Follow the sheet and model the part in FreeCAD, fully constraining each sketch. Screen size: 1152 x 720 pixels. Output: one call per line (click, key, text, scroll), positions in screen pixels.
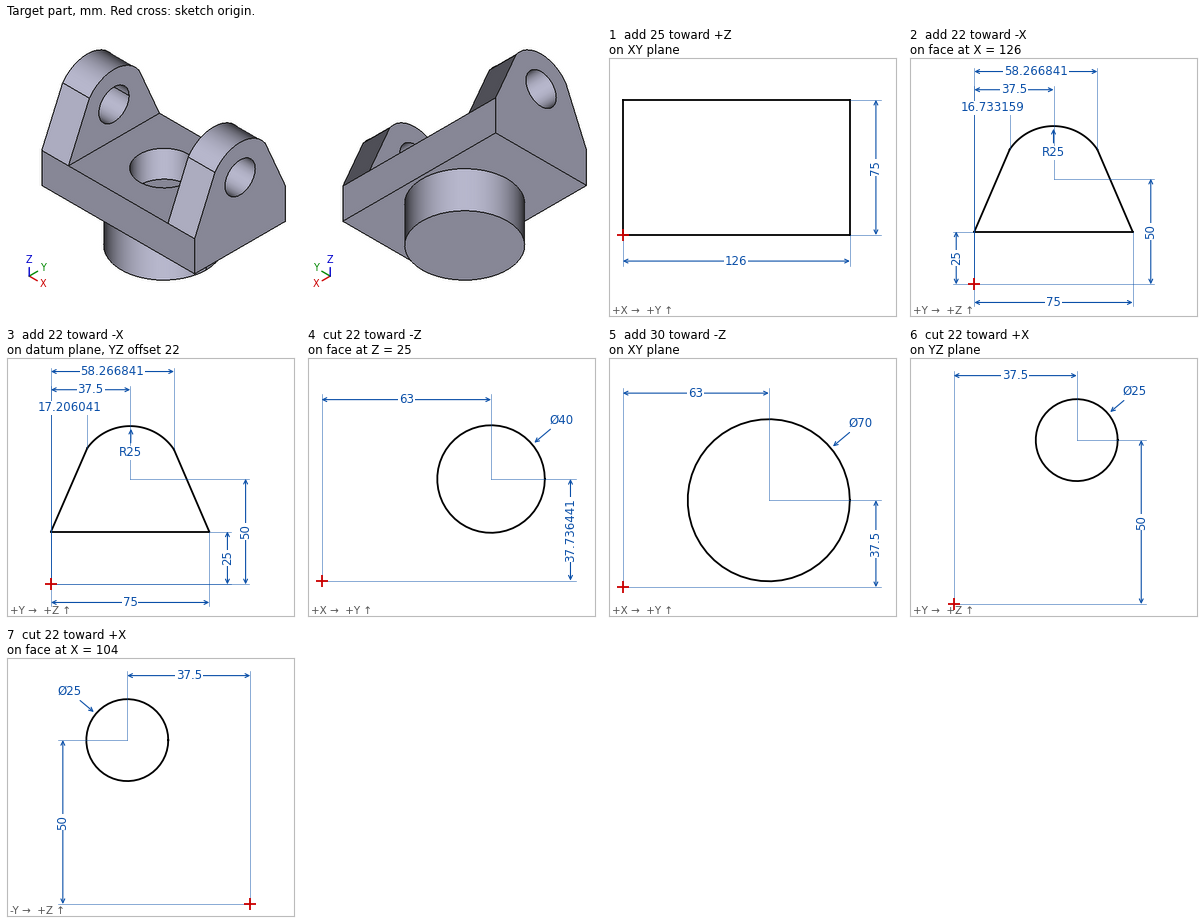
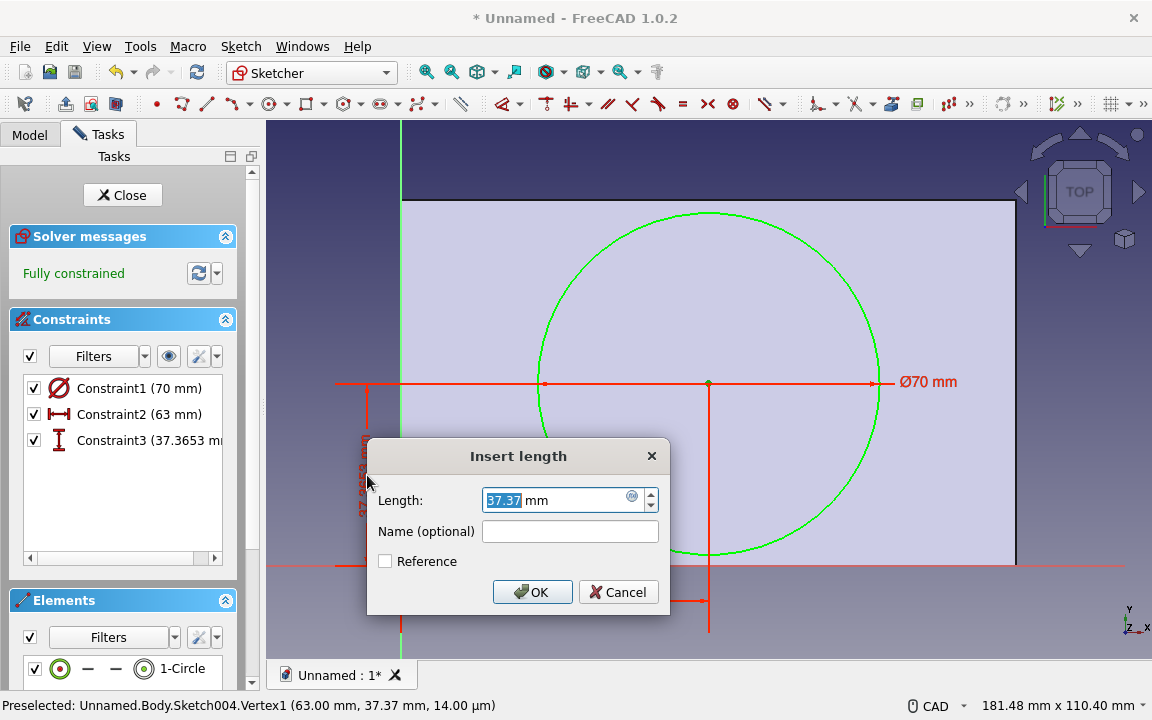
text(37.5)
key(Return)
key(Escape)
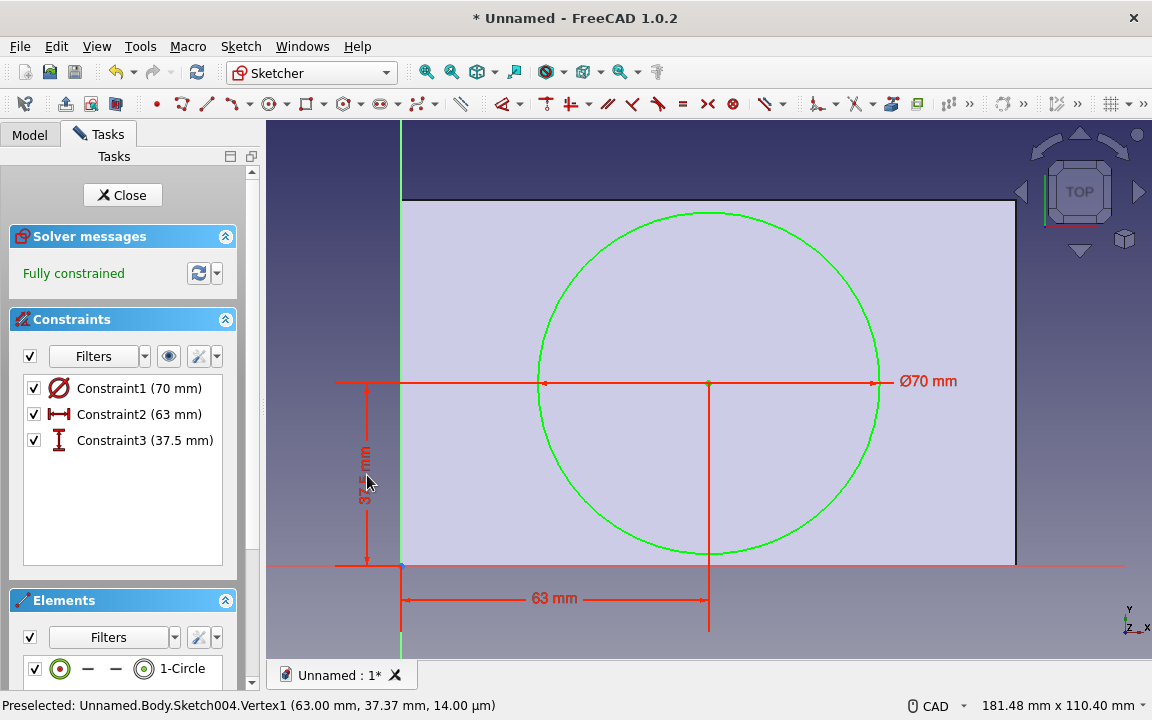
click(123, 195)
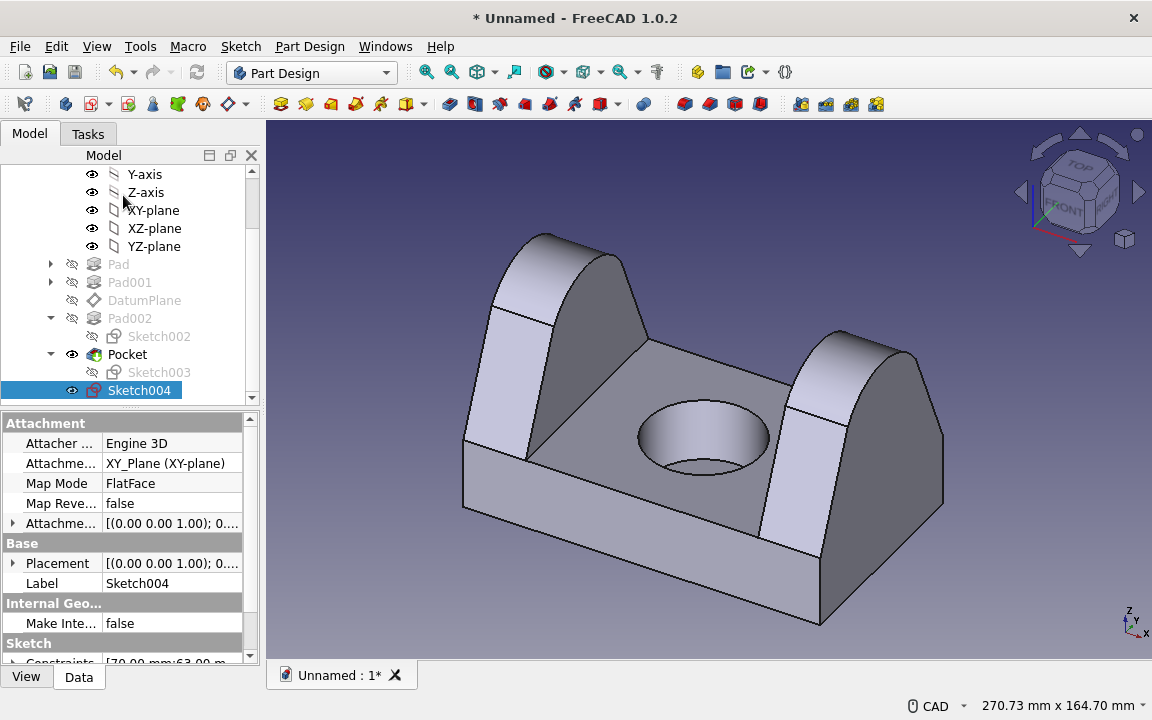
click(281, 104)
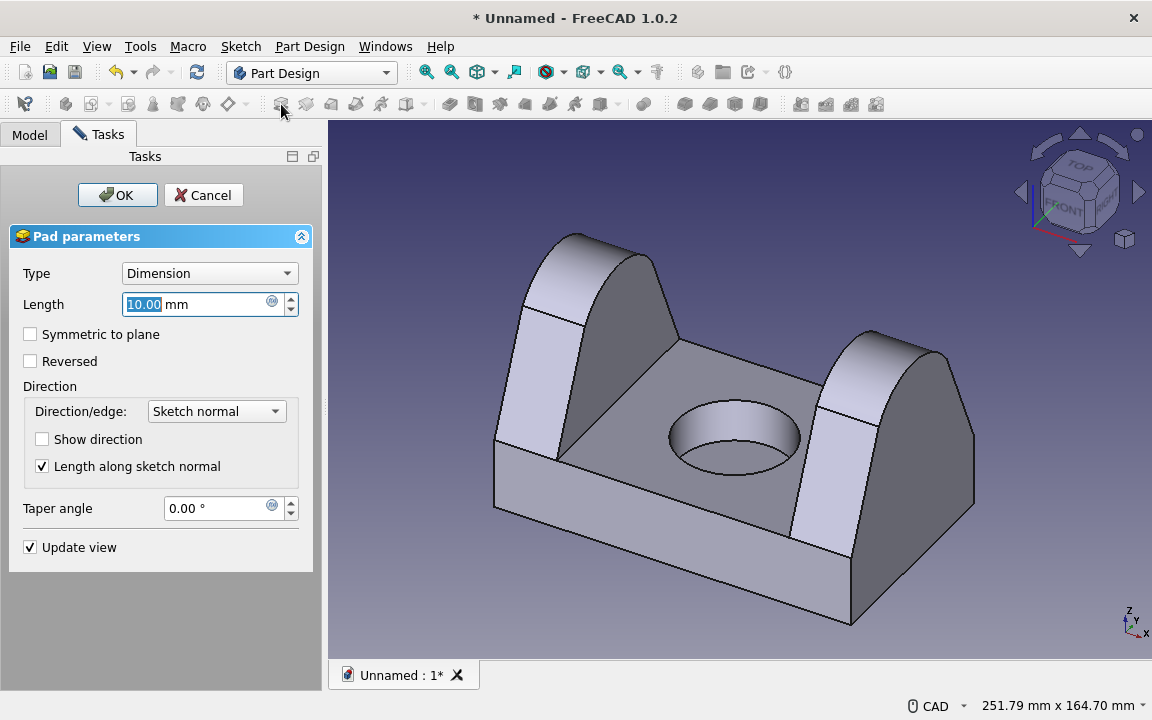
text(30)
key(Tab)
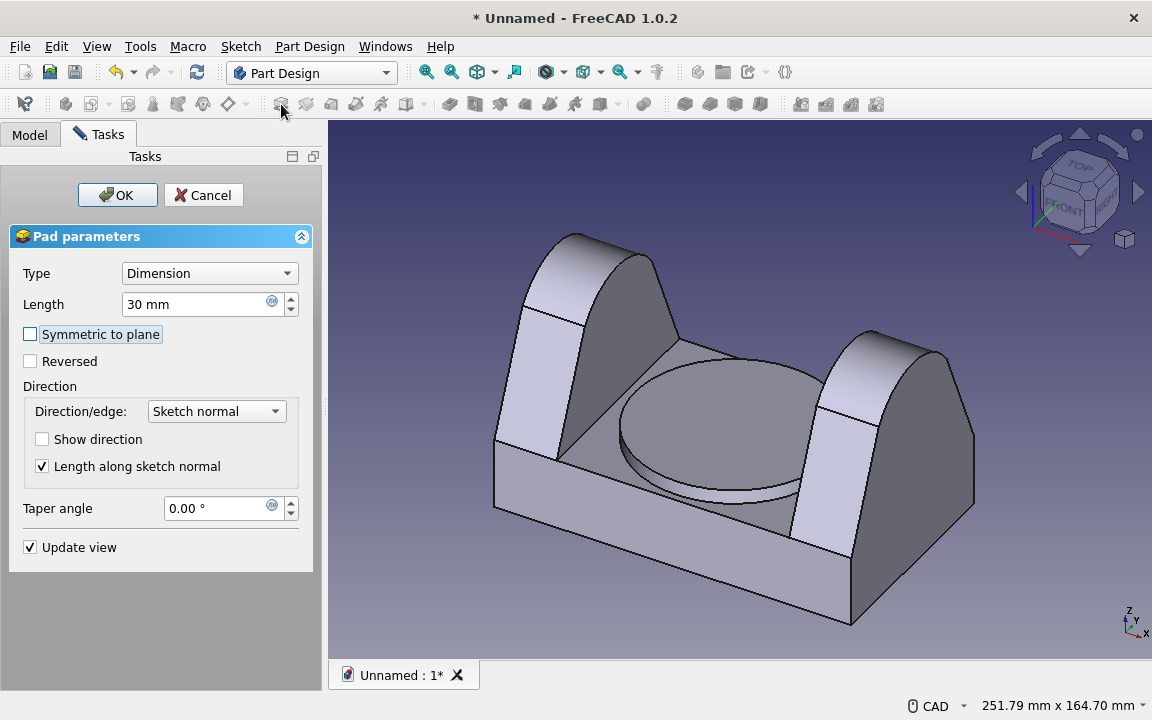
click(31, 361)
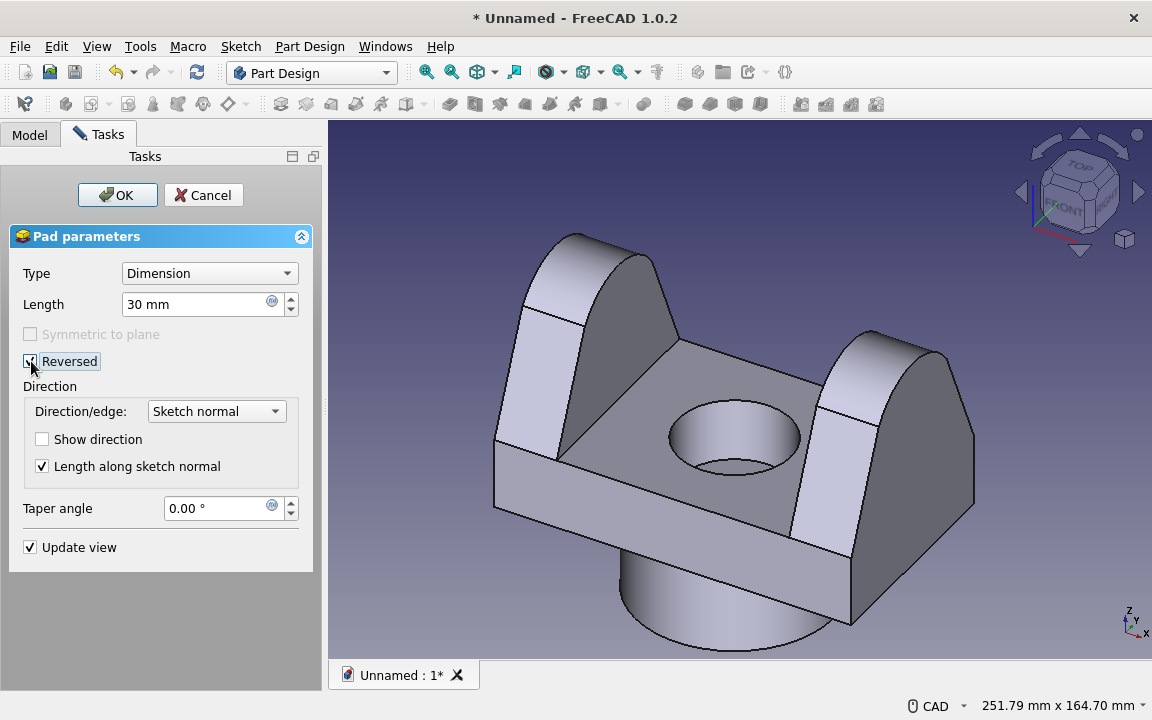
click(118, 195)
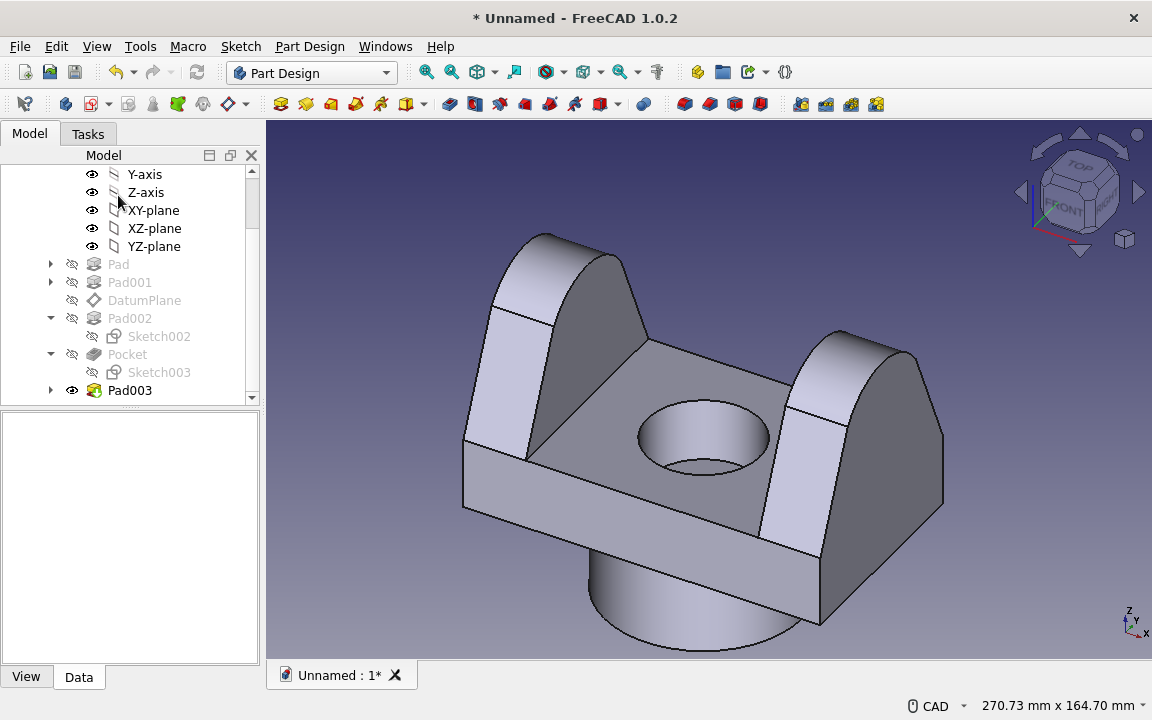
click(427, 72)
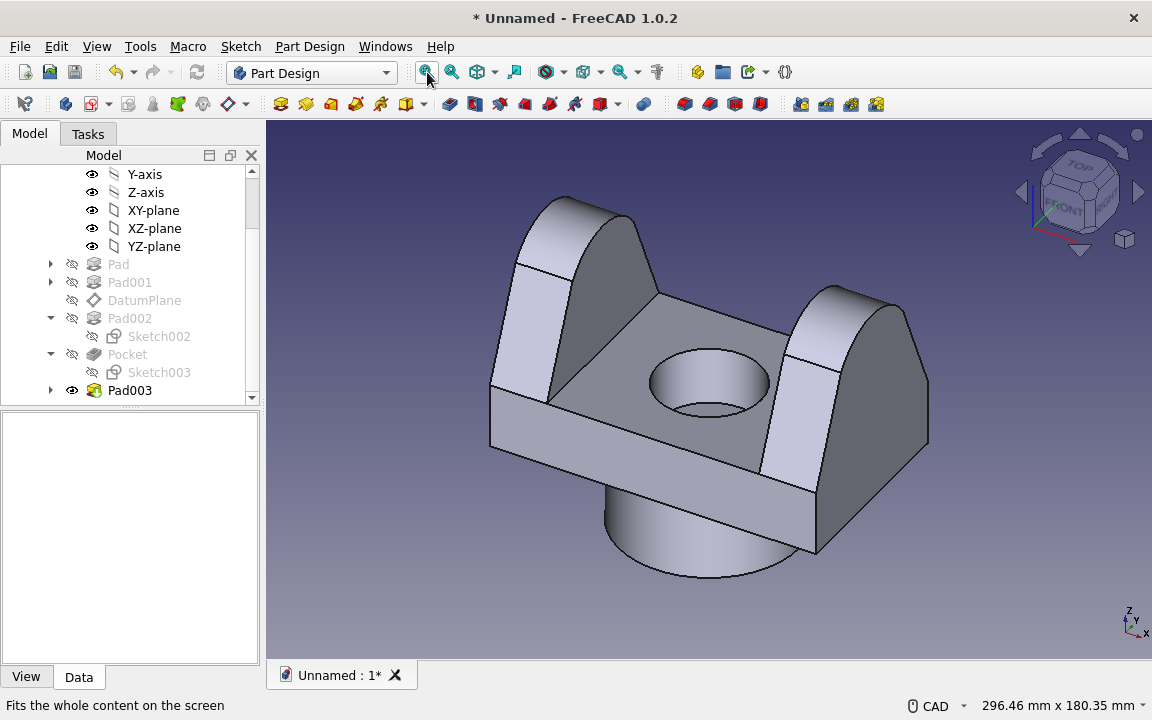
click(90, 104)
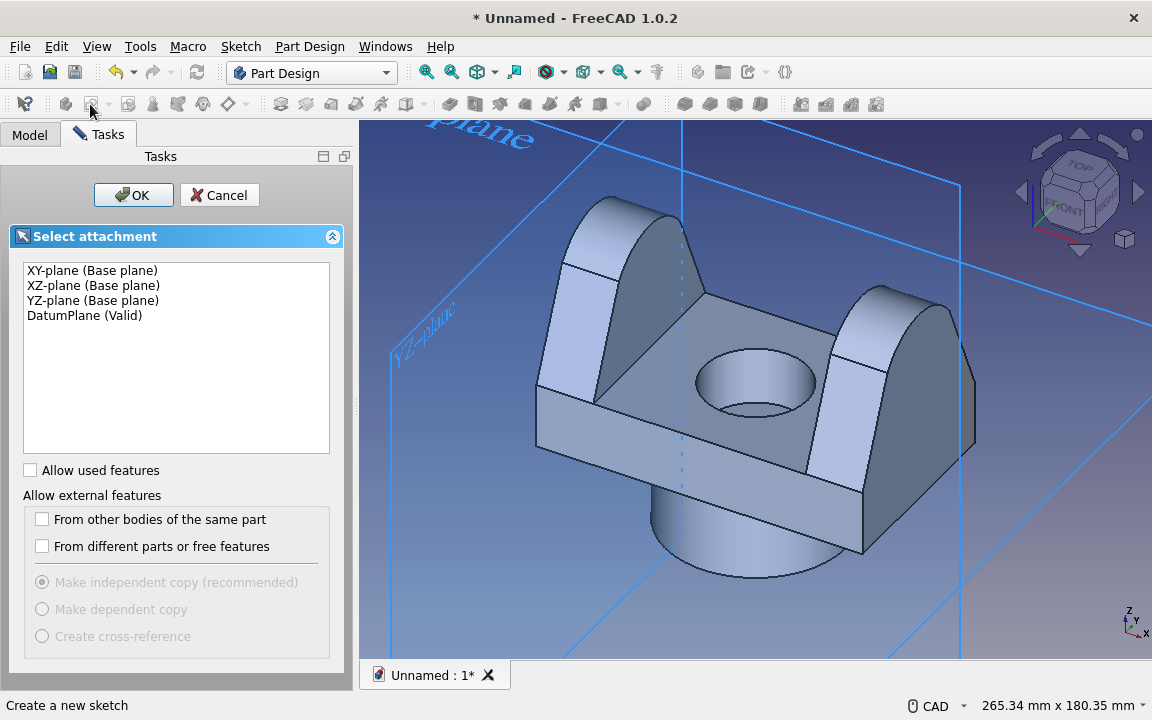
click(84, 300)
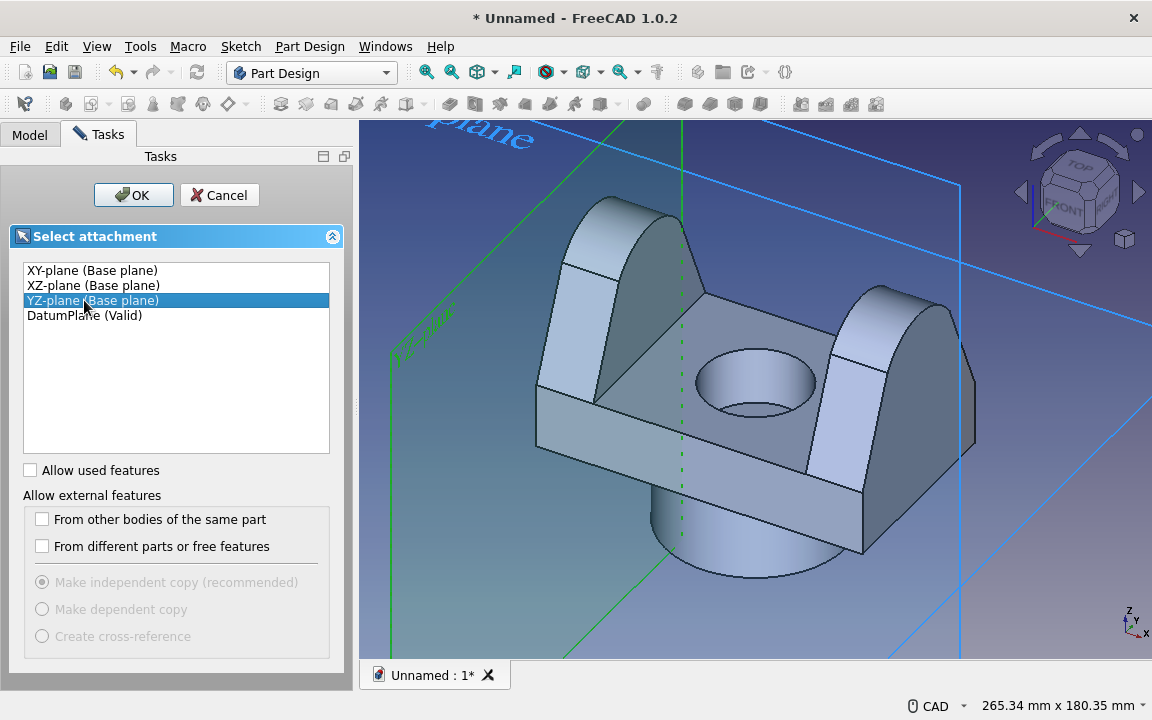
click(134, 195)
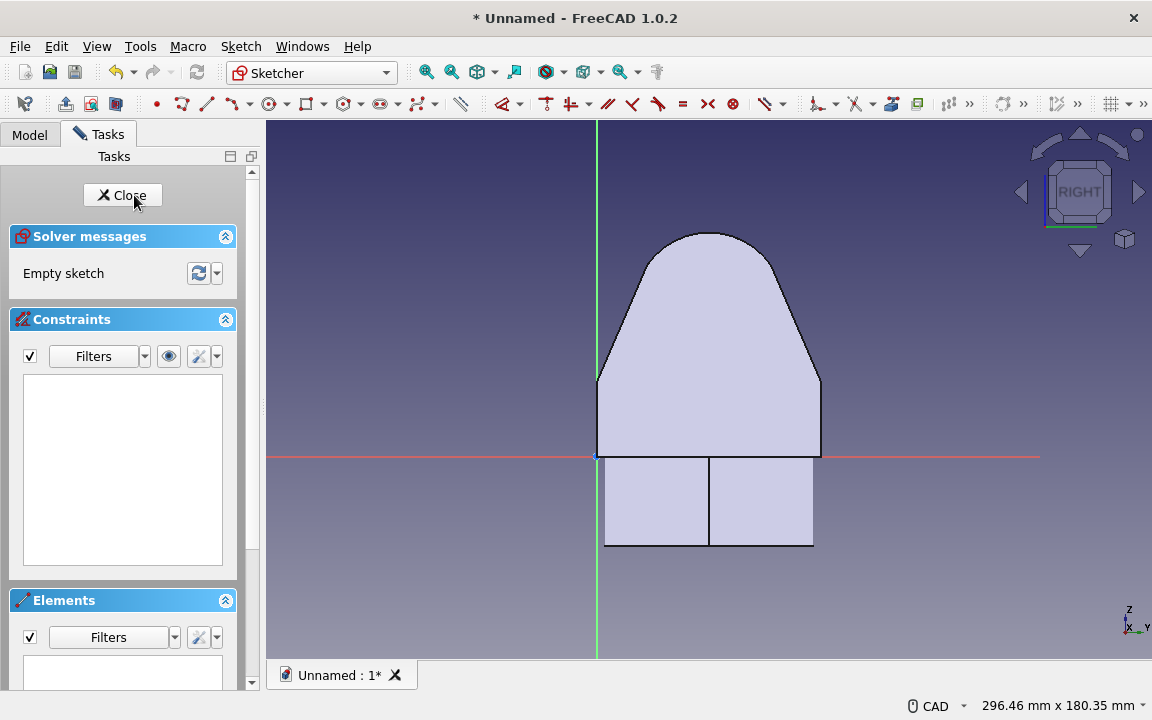
click(116, 104)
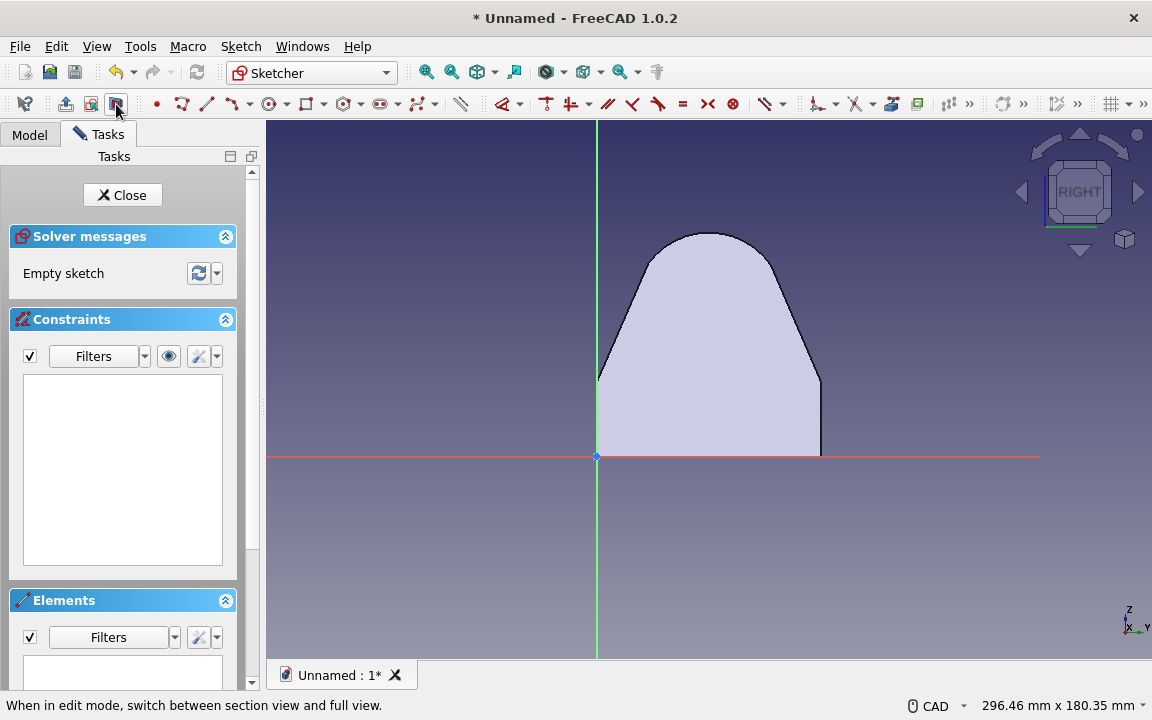
scroll(726, 287, up, 8)